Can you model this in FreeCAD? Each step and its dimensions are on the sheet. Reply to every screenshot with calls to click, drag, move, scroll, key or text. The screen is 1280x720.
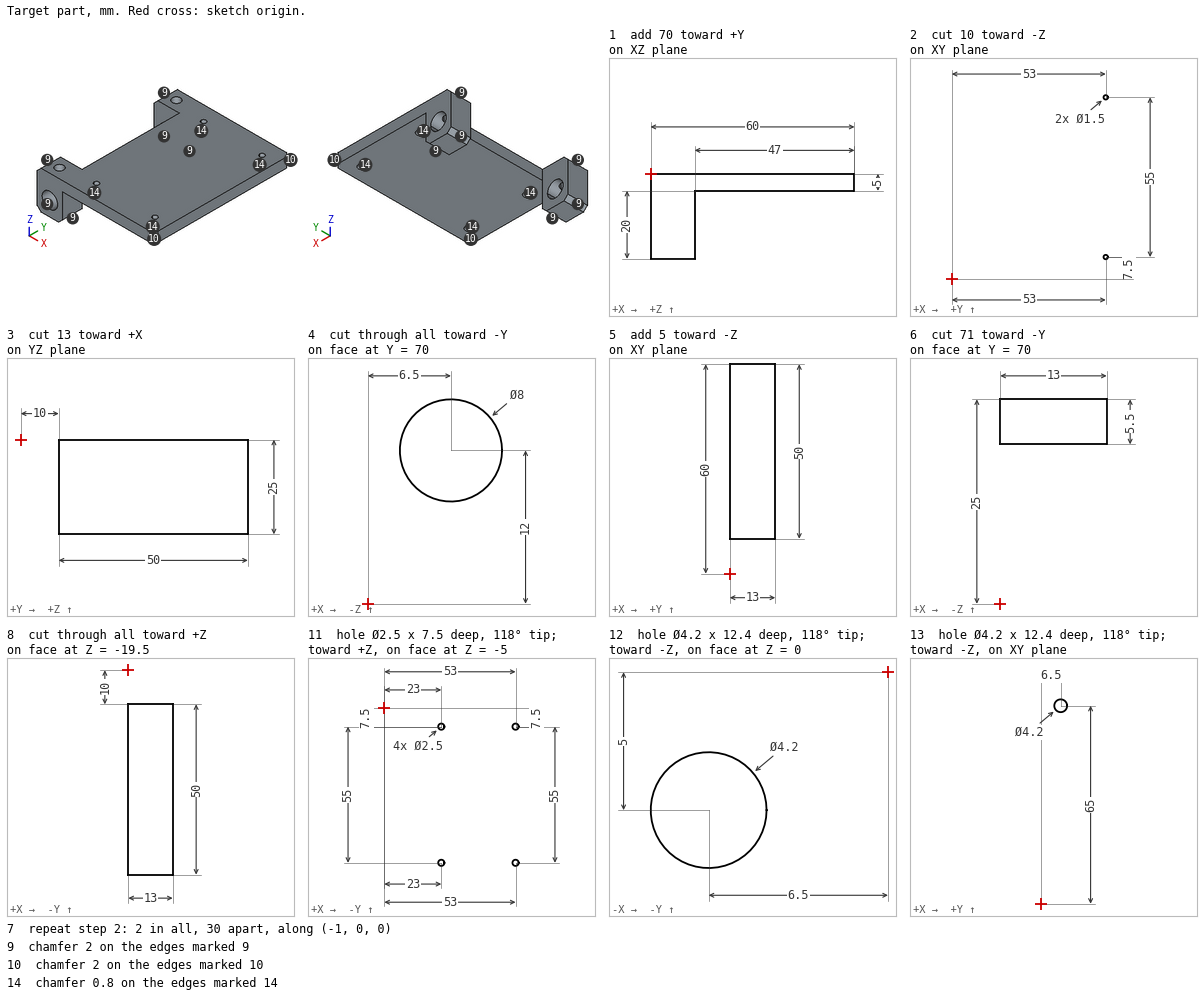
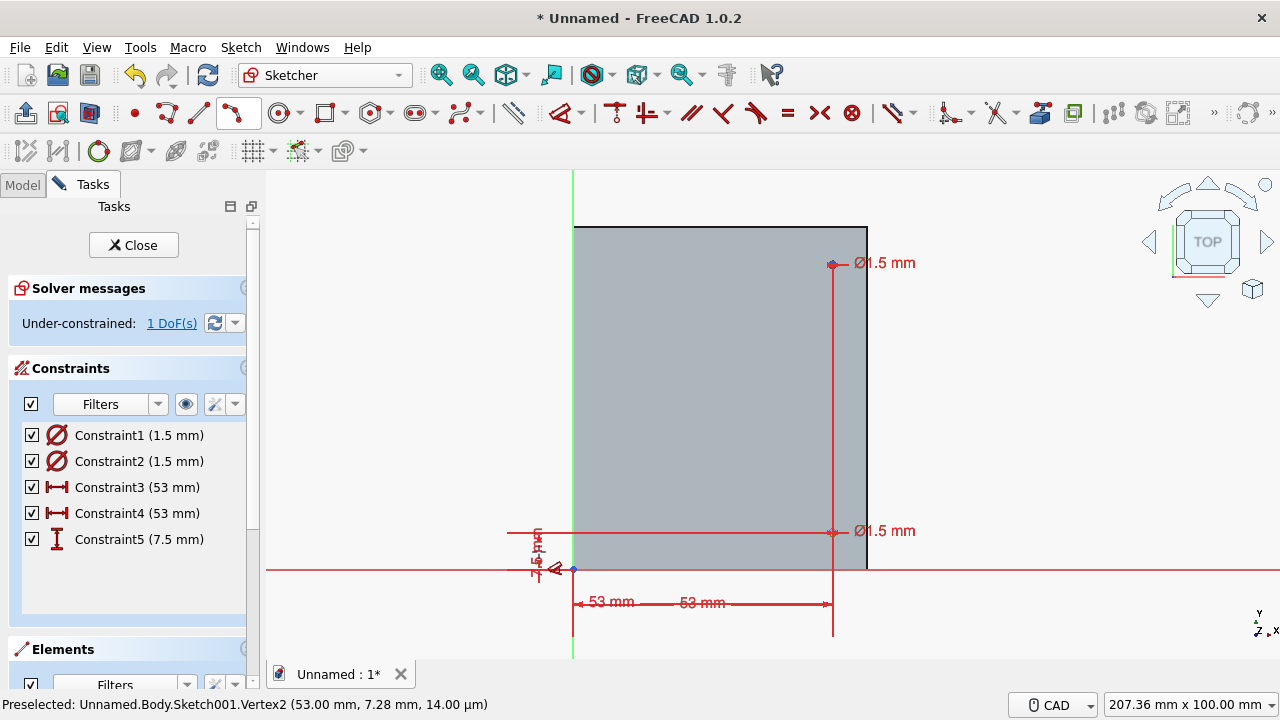
click(833, 265)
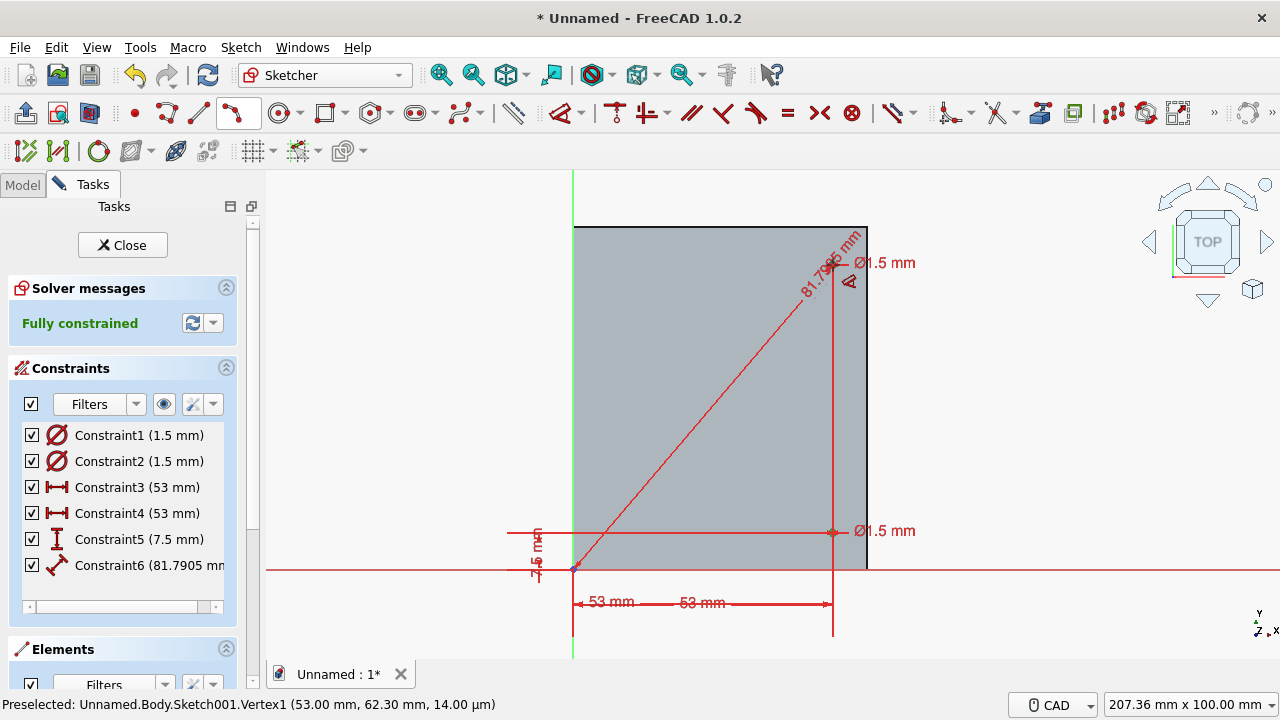
click(833, 533)
click(867, 399)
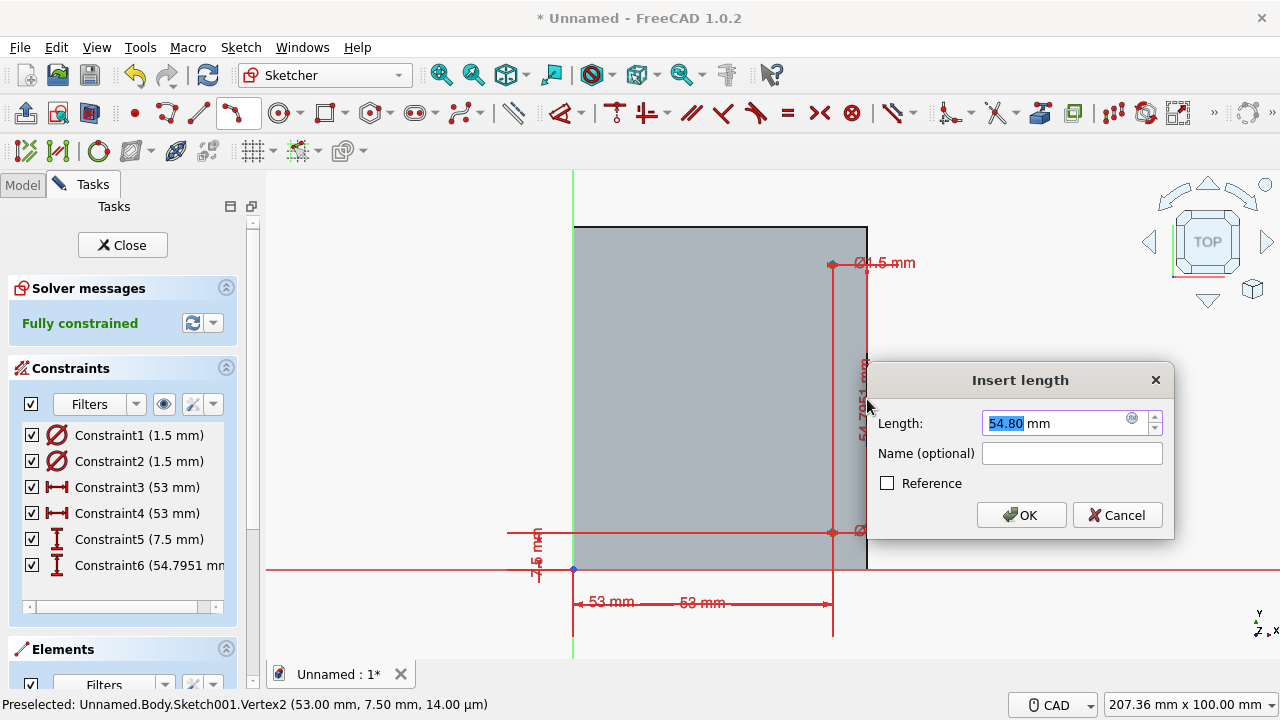
text(55)
key(Return)
key(Escape)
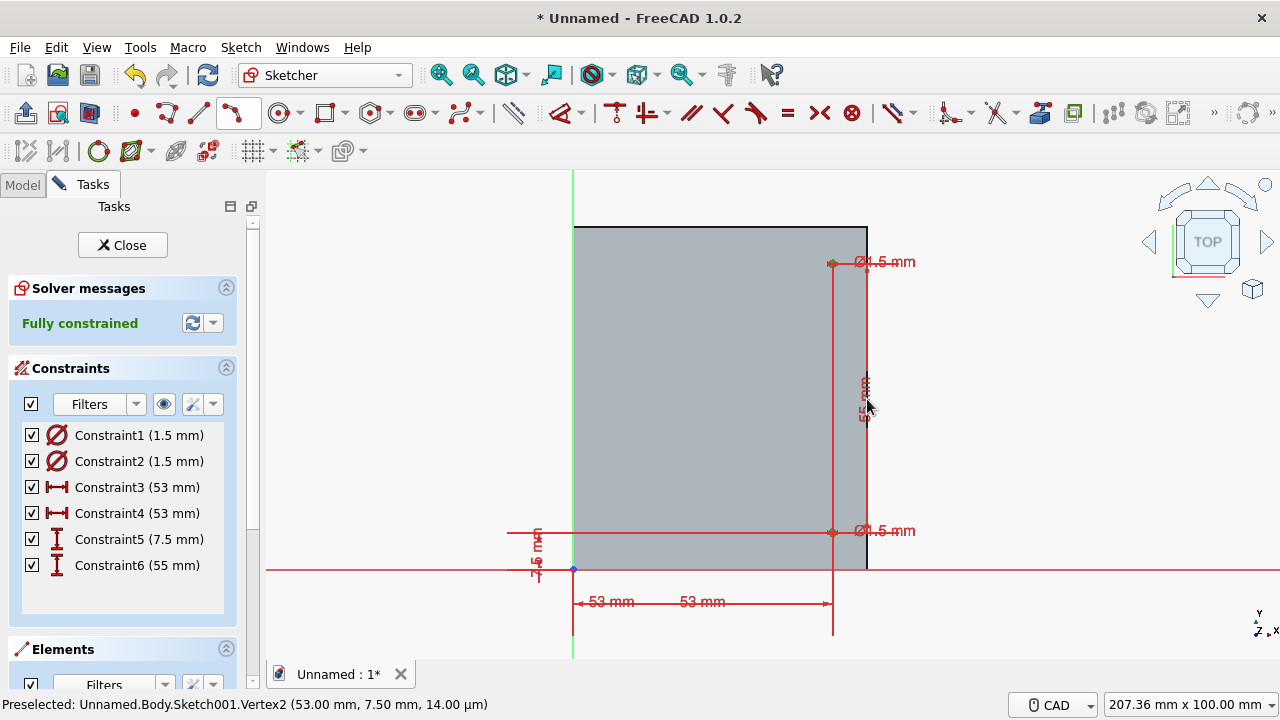
click(123, 245)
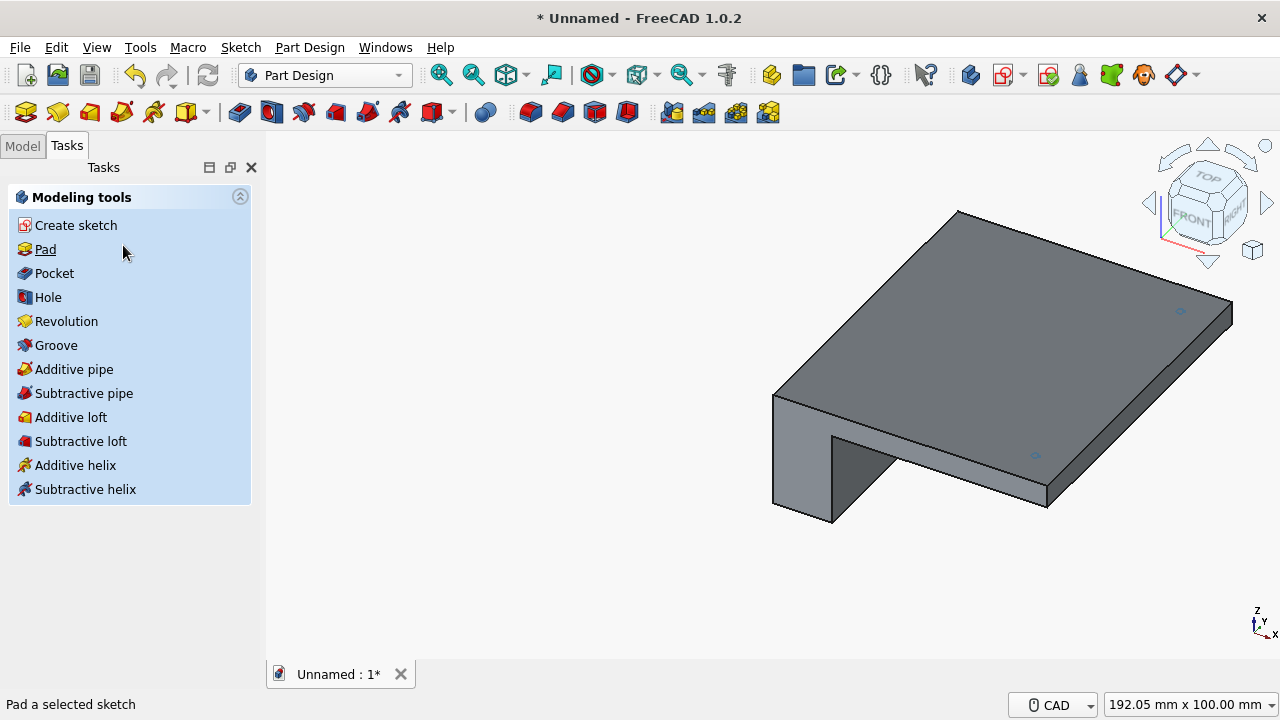
click(240, 112)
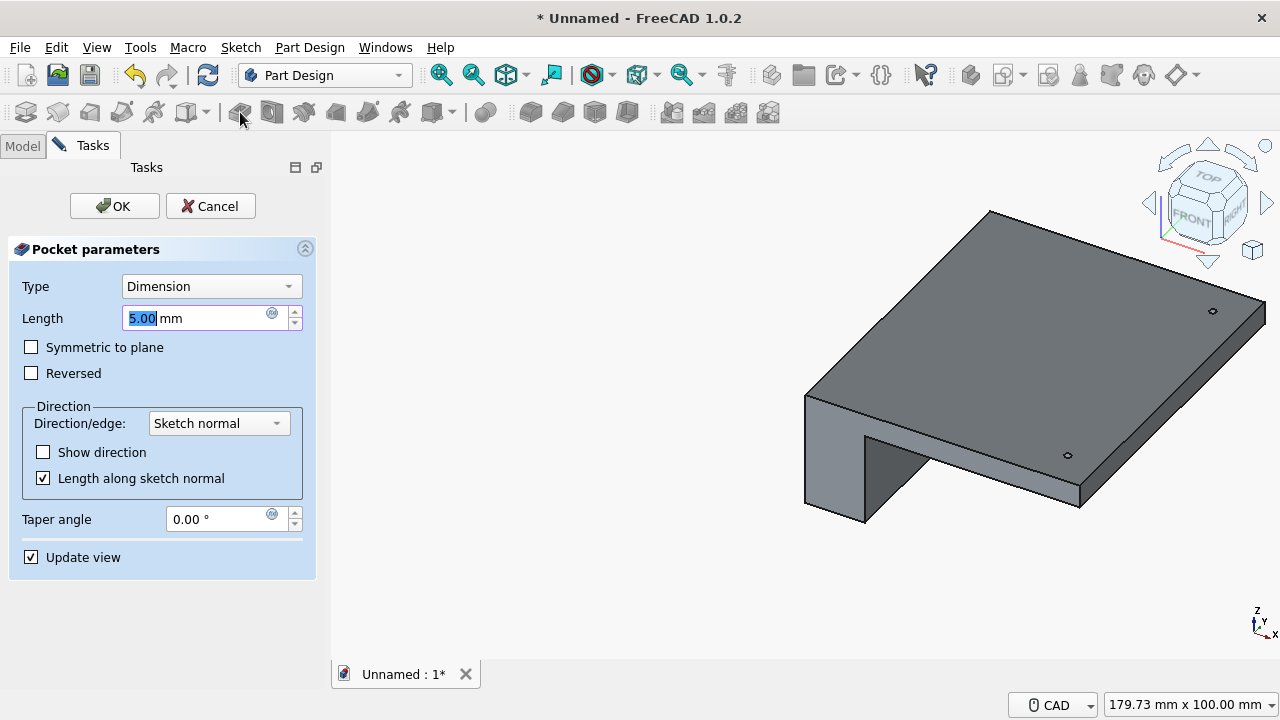
text(10)
key(Tab)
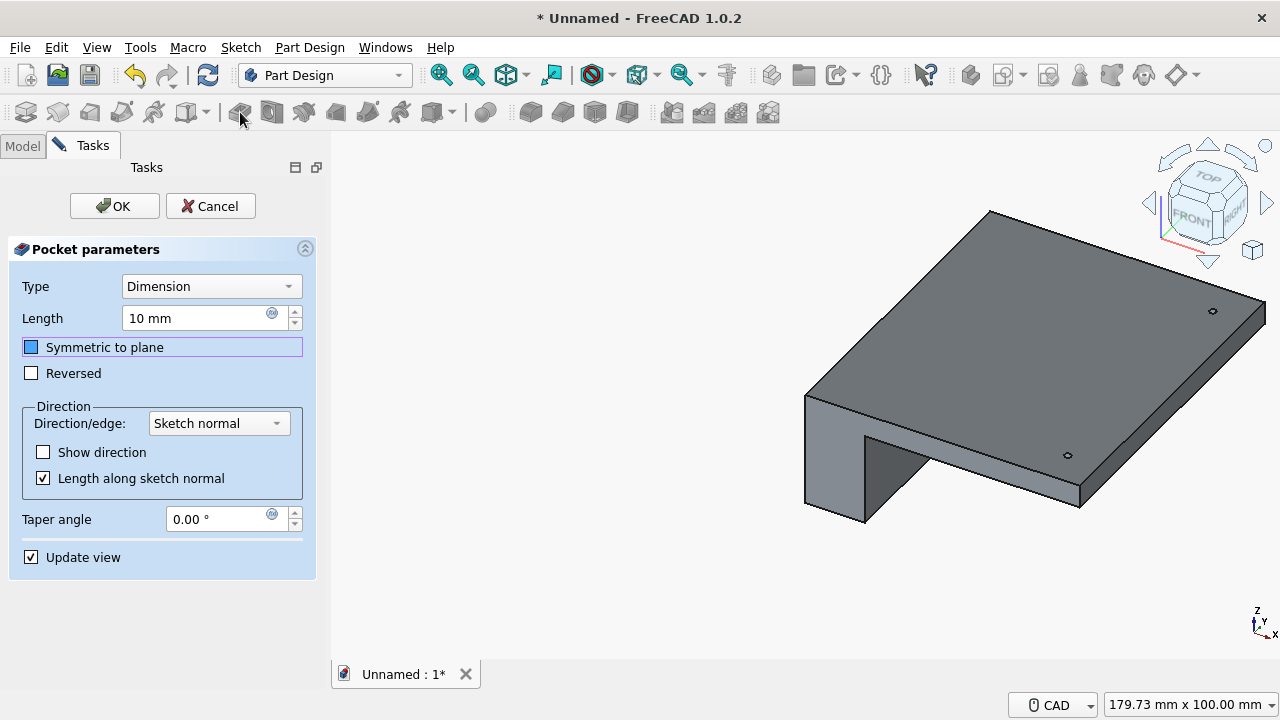
click(115, 206)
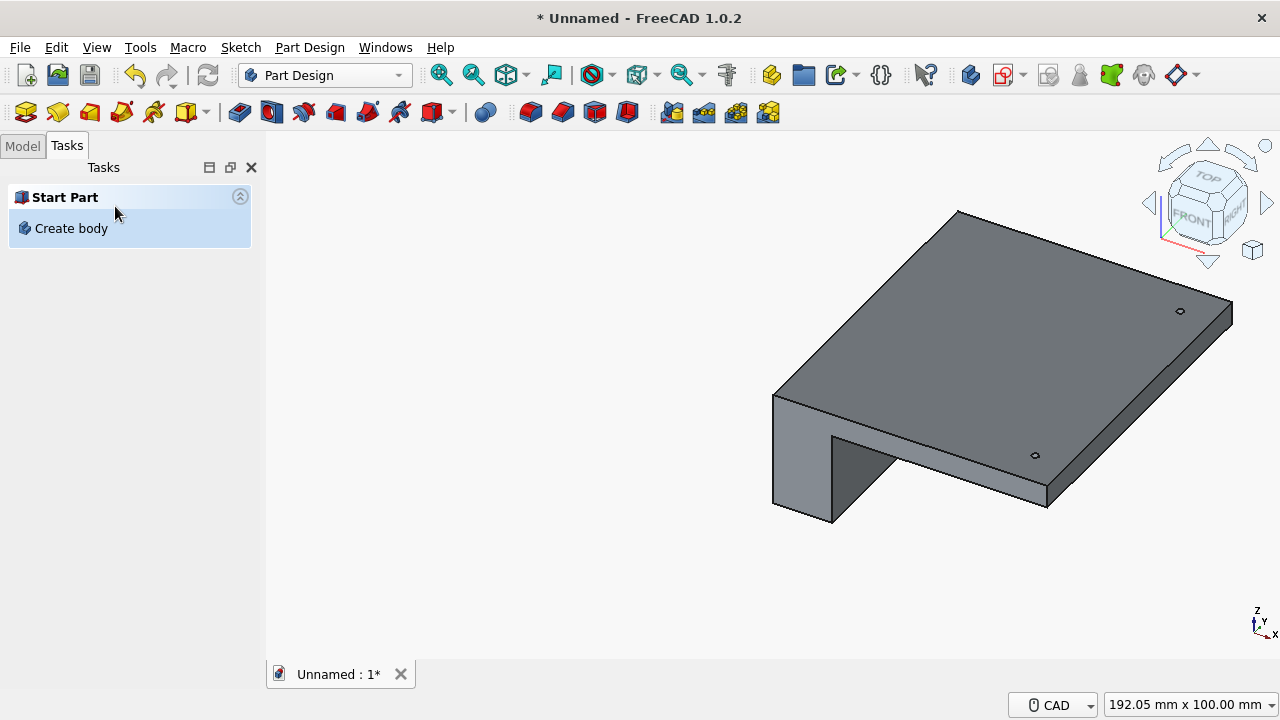
click(1004, 76)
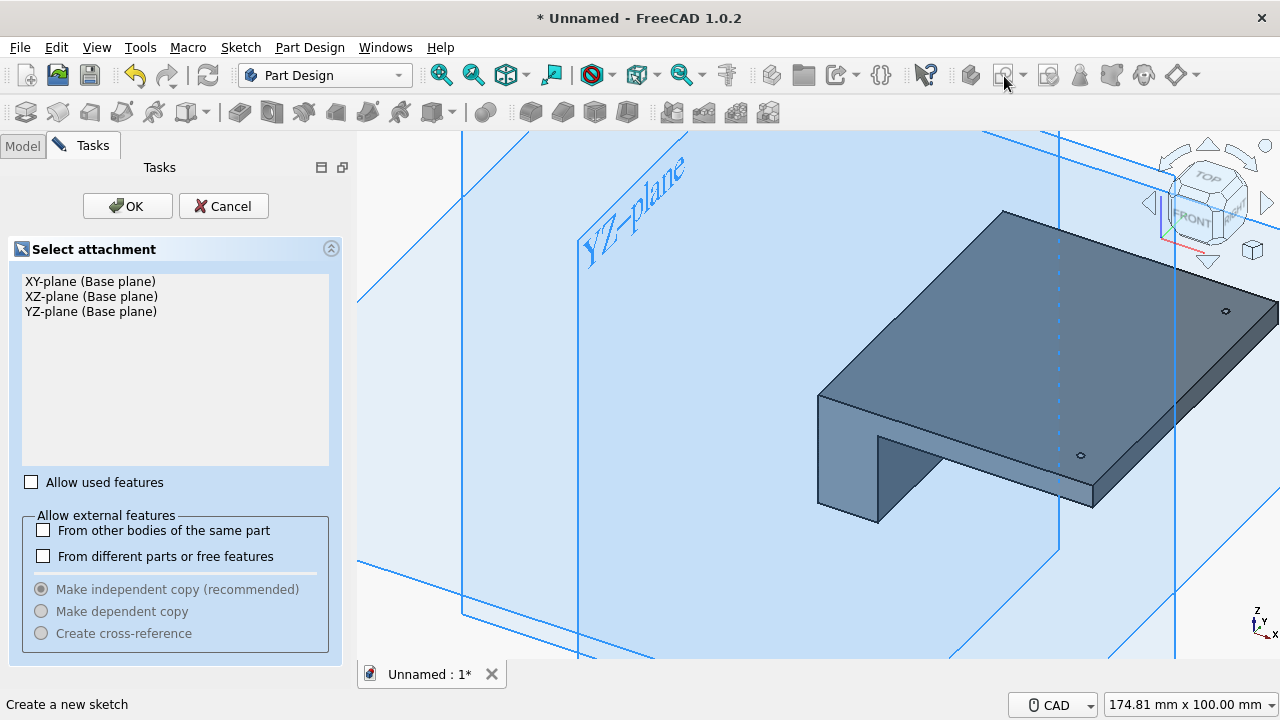
click(82, 312)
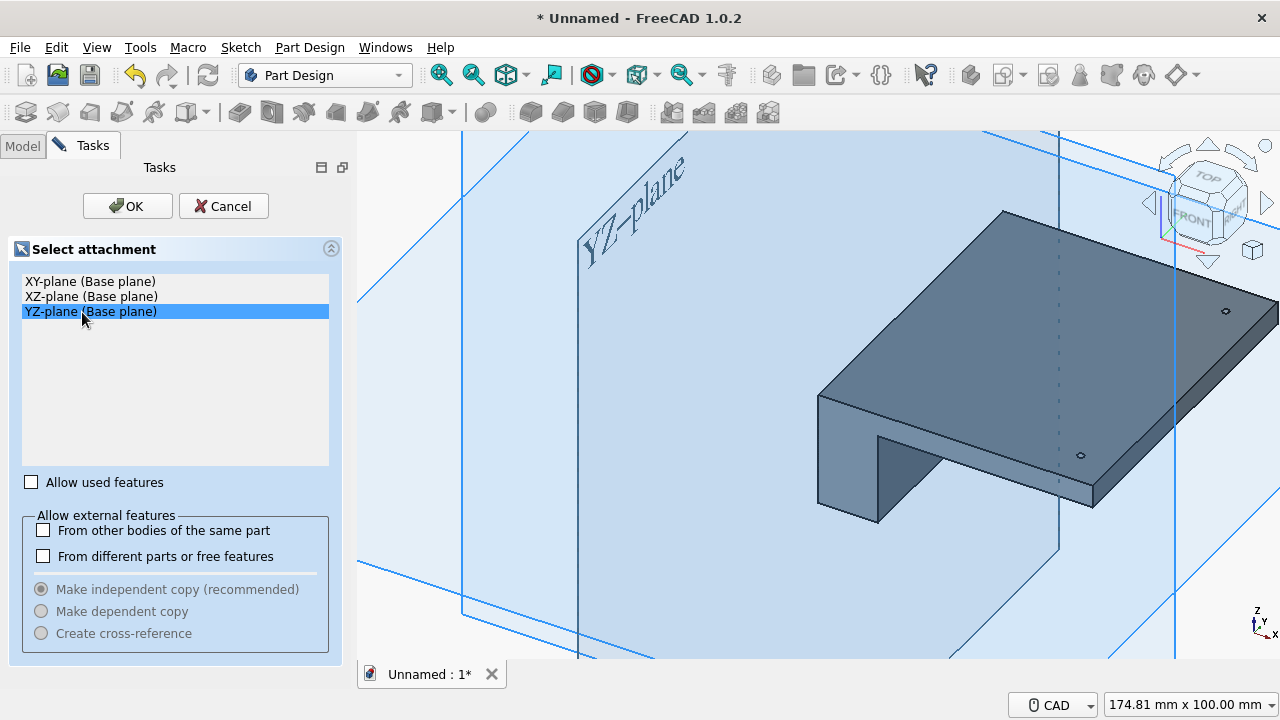
click(128, 206)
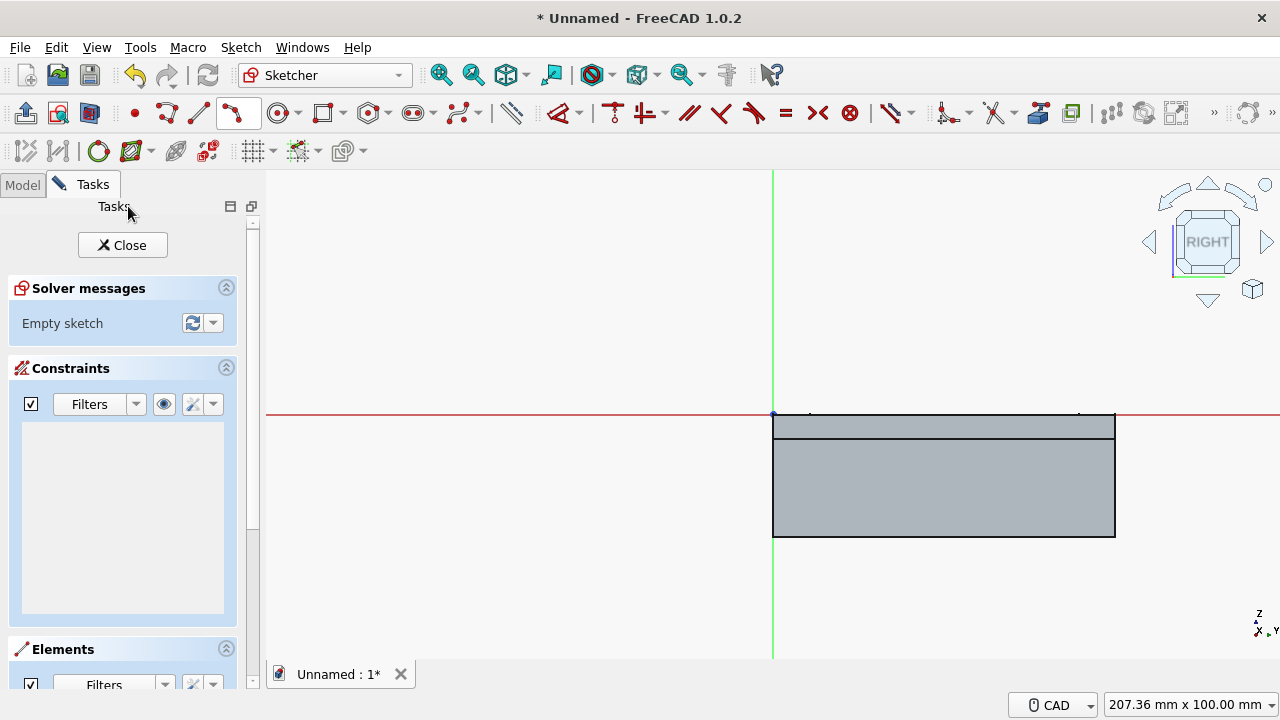
key(q)
key(s)